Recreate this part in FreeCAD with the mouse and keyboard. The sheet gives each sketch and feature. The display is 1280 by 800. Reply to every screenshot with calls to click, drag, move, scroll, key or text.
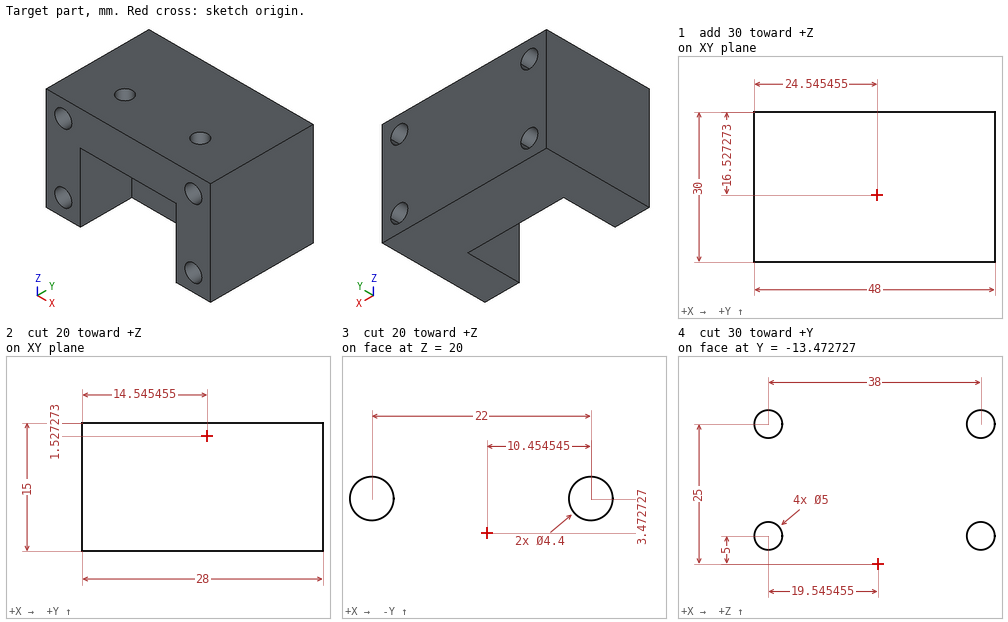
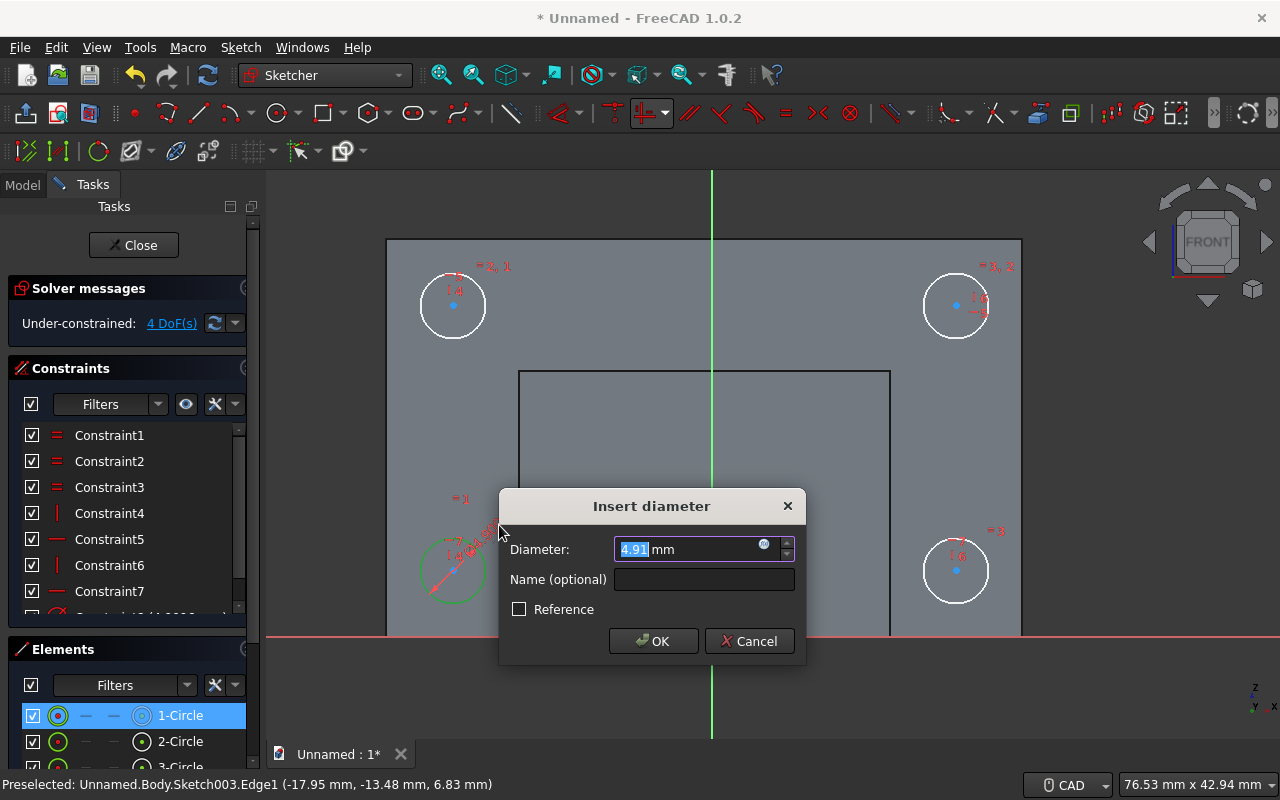
text(5)
key(Return)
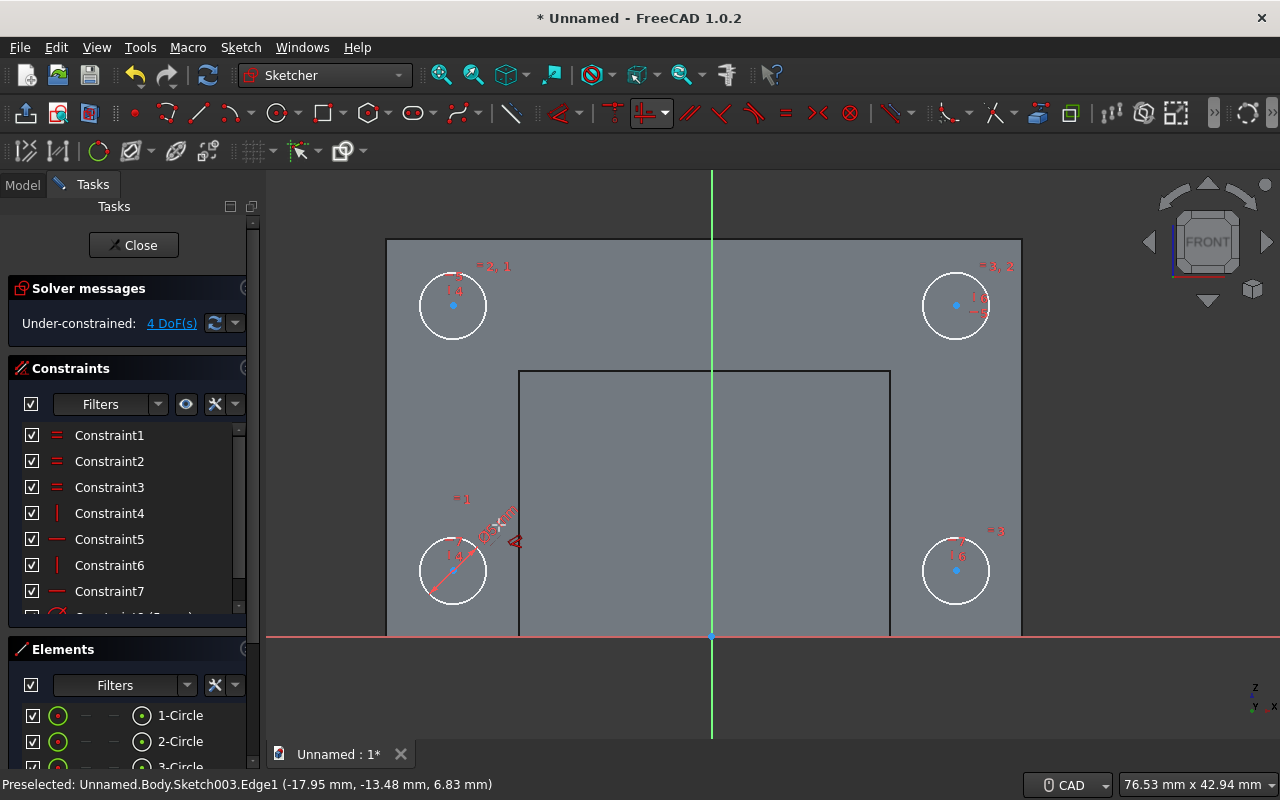
click(453, 571)
click(419, 604)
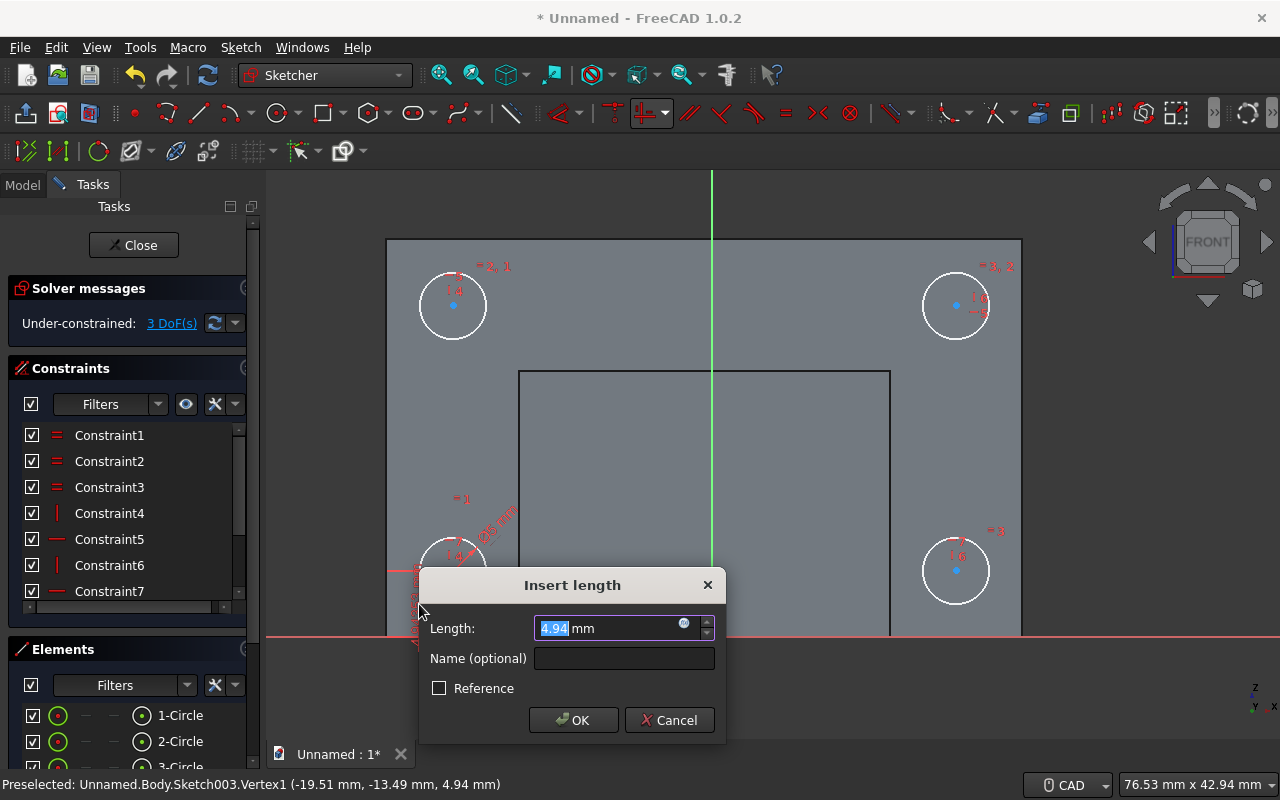
text(5)
key(Return)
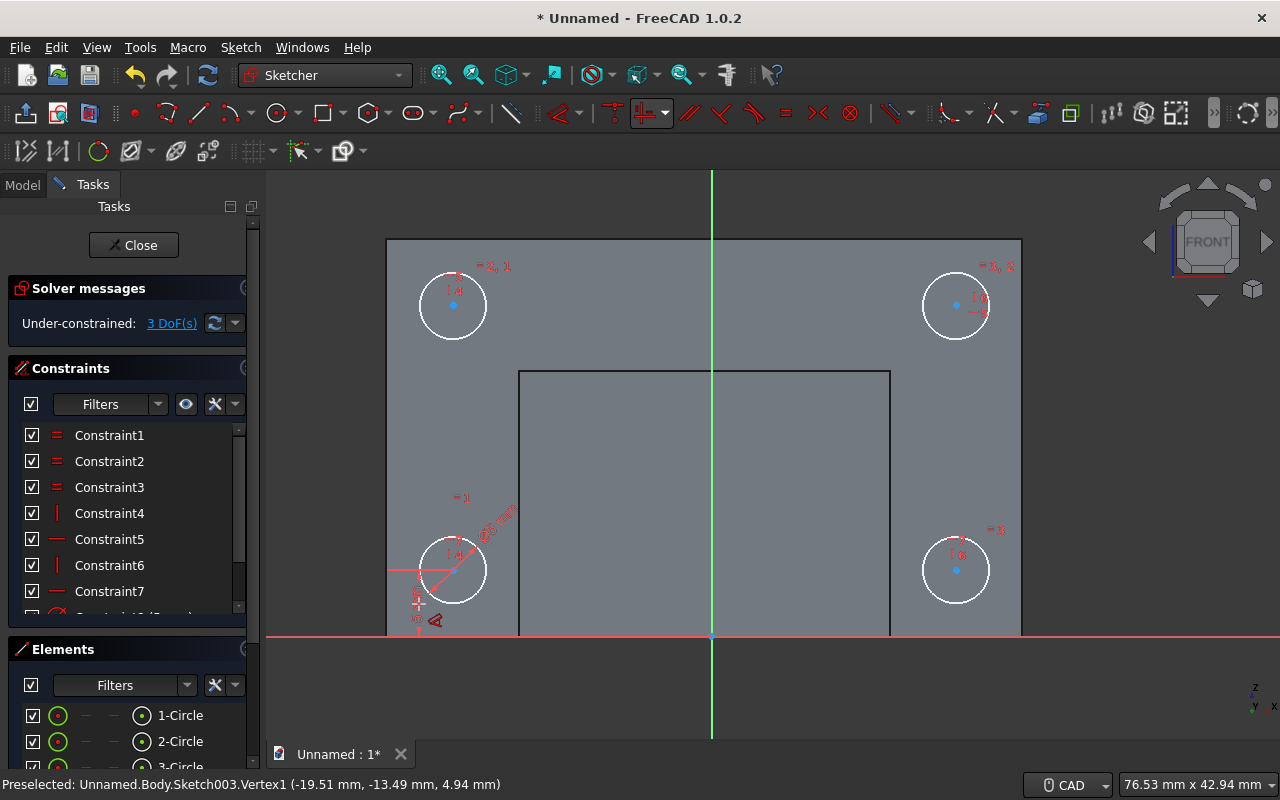
click(453, 306)
click(419, 471)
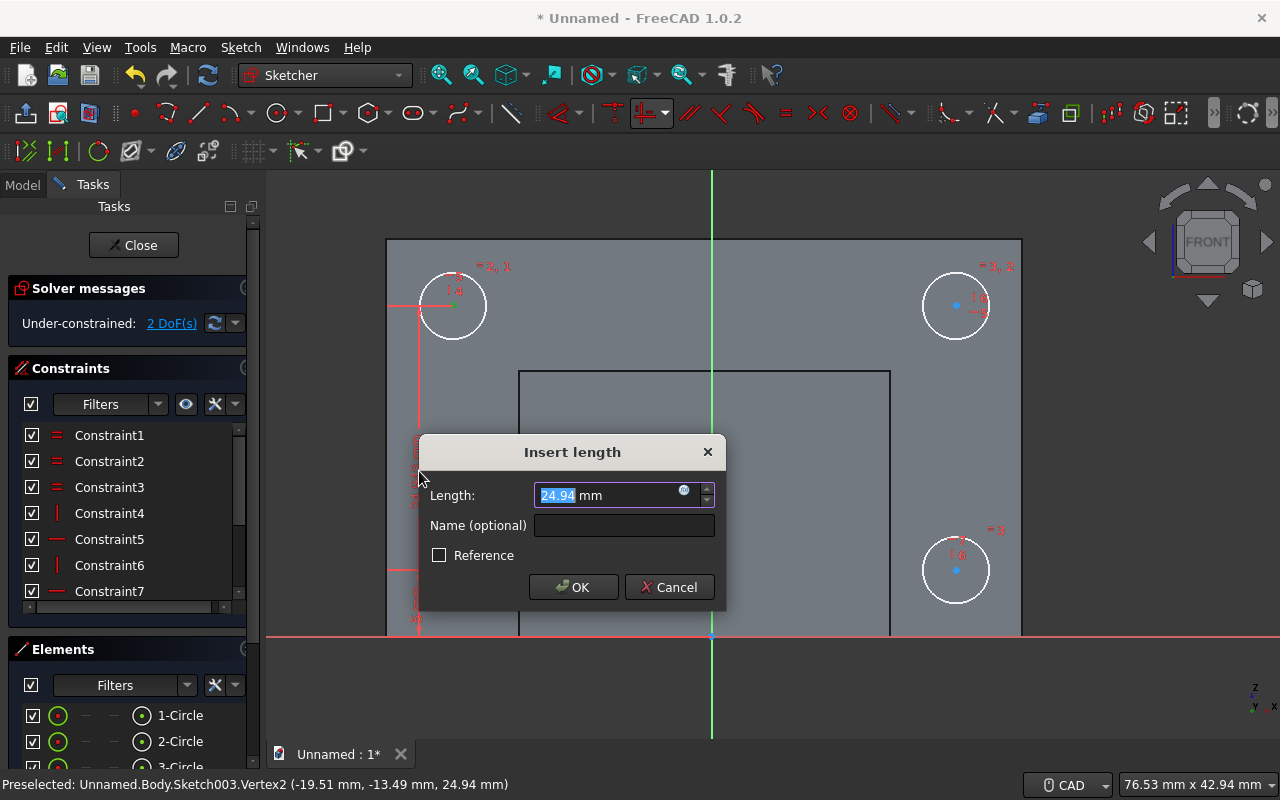
text(25)
key(Return)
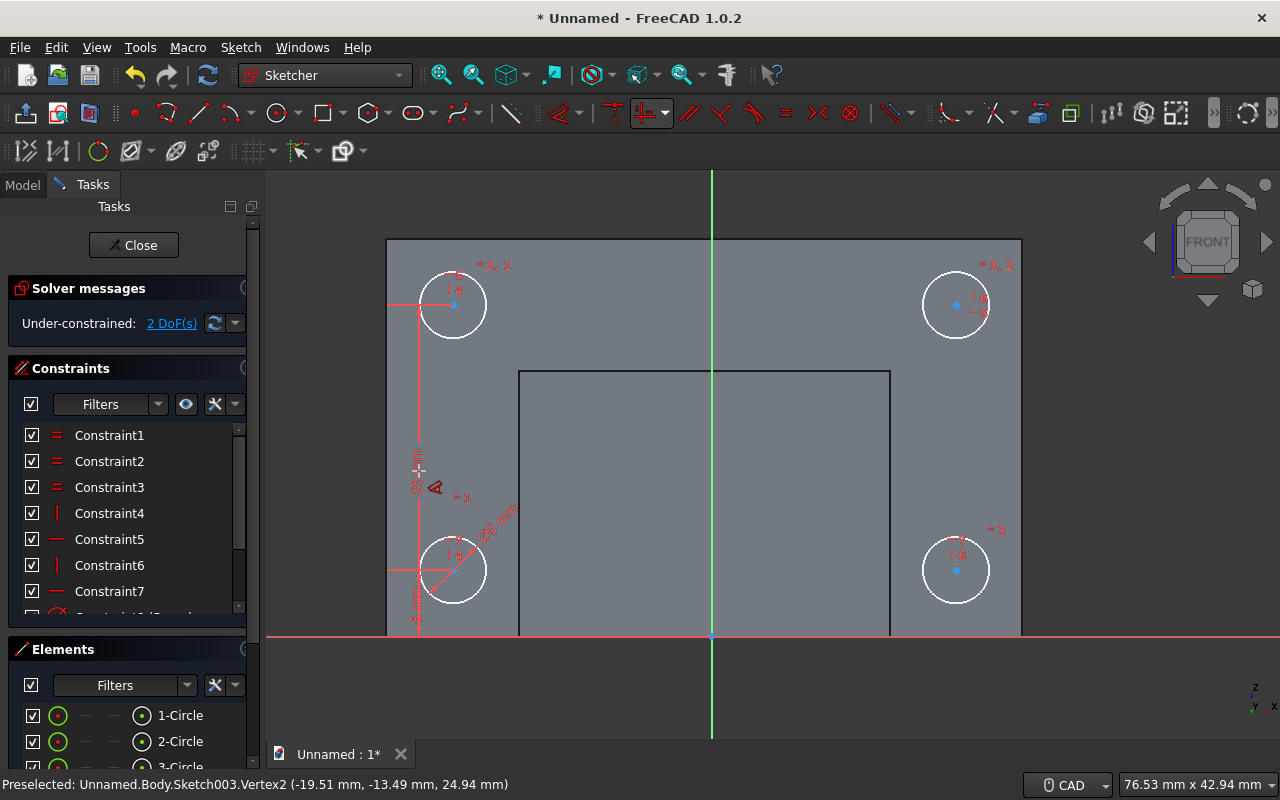
click(453, 305)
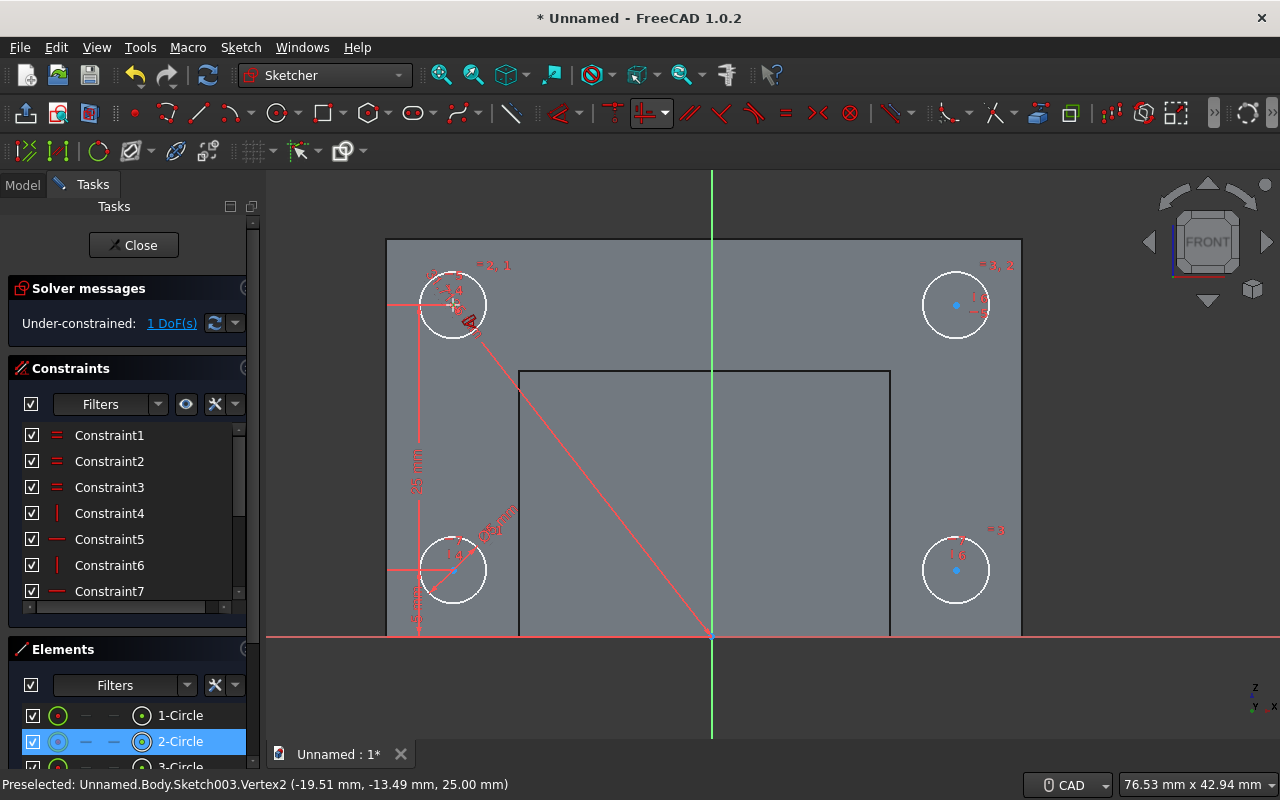
click(956, 305)
click(589, 271)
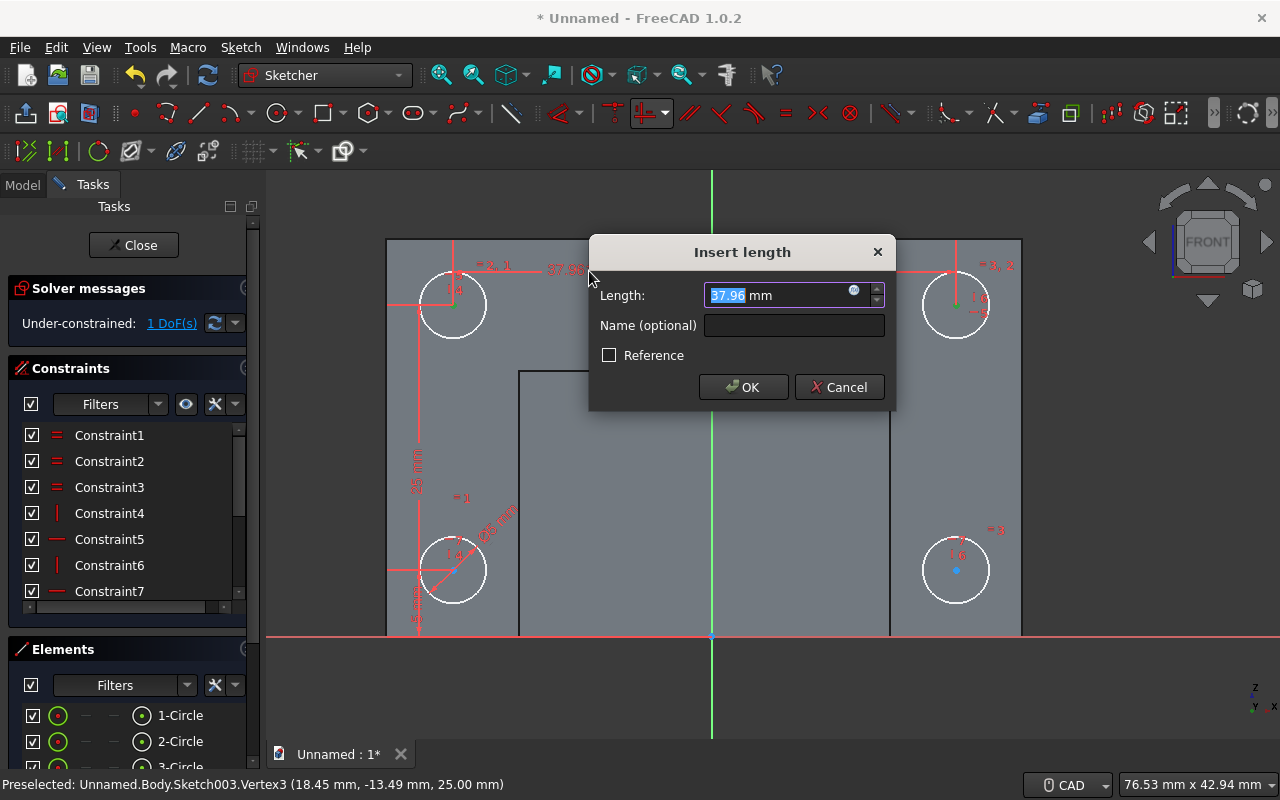
text(38)
key(Return)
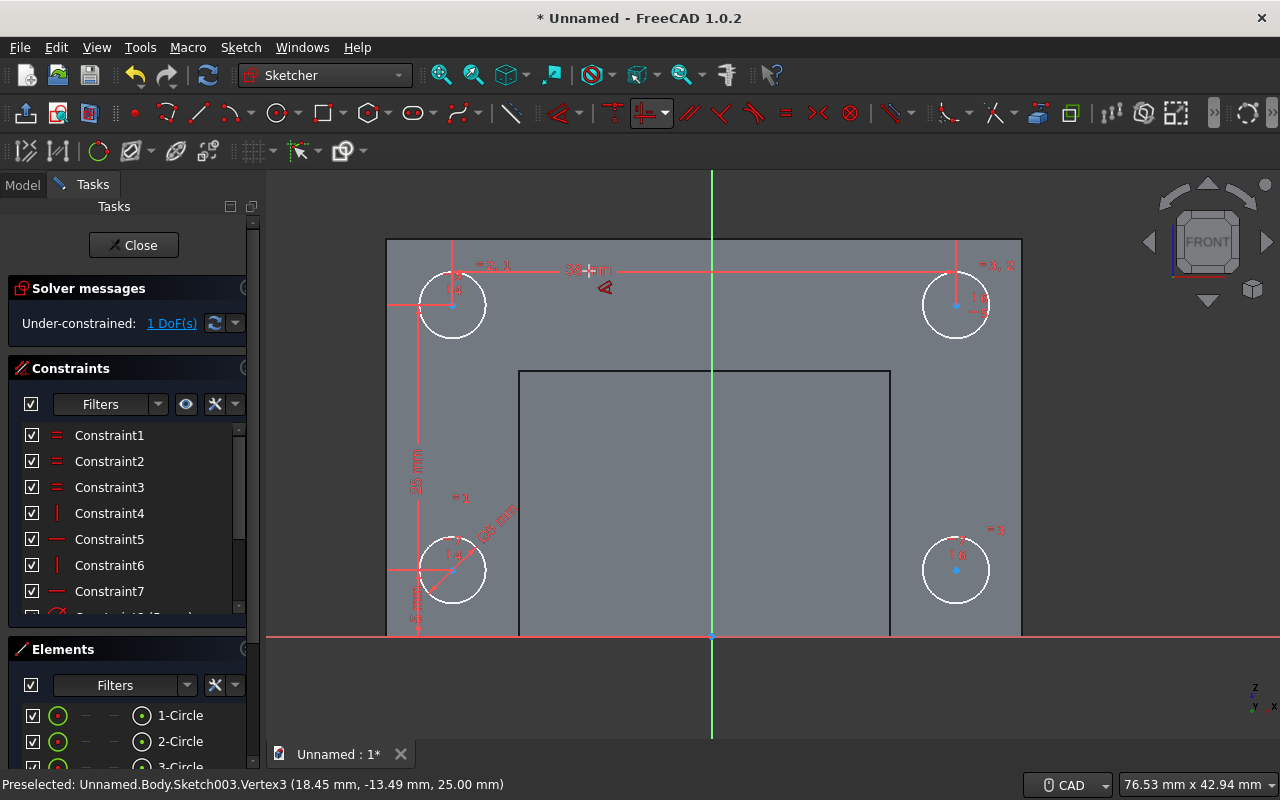
click(452, 570)
click(582, 671)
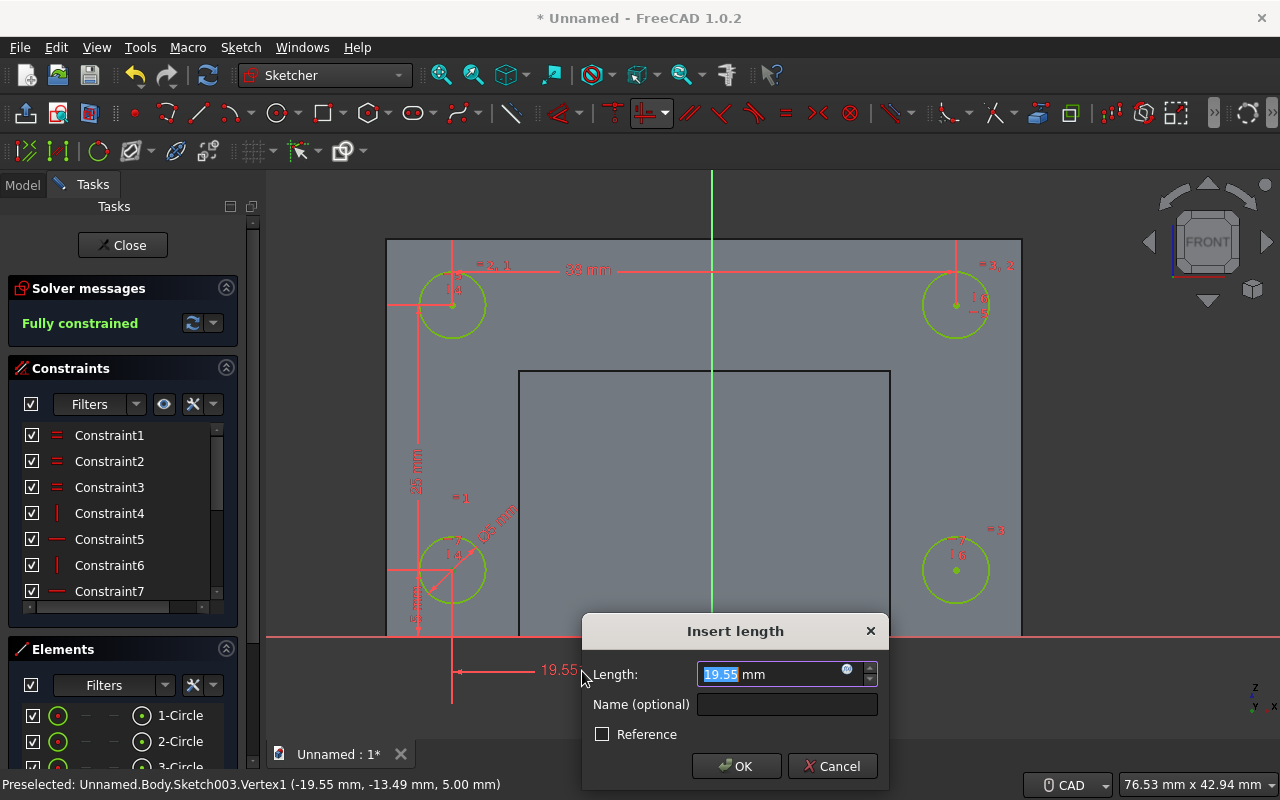
text(19.545455)
key(Return)
key(Escape)